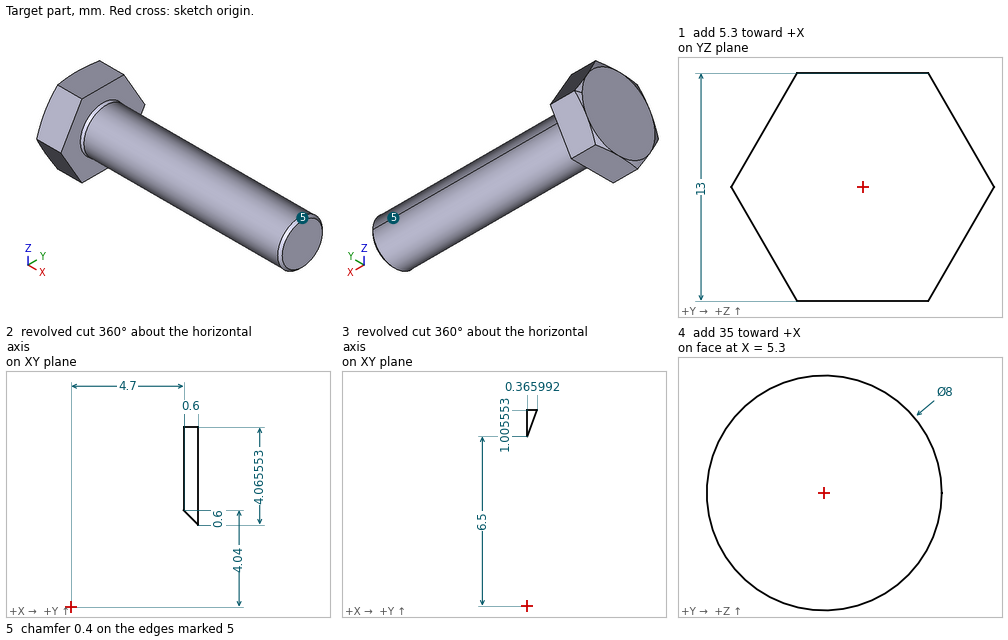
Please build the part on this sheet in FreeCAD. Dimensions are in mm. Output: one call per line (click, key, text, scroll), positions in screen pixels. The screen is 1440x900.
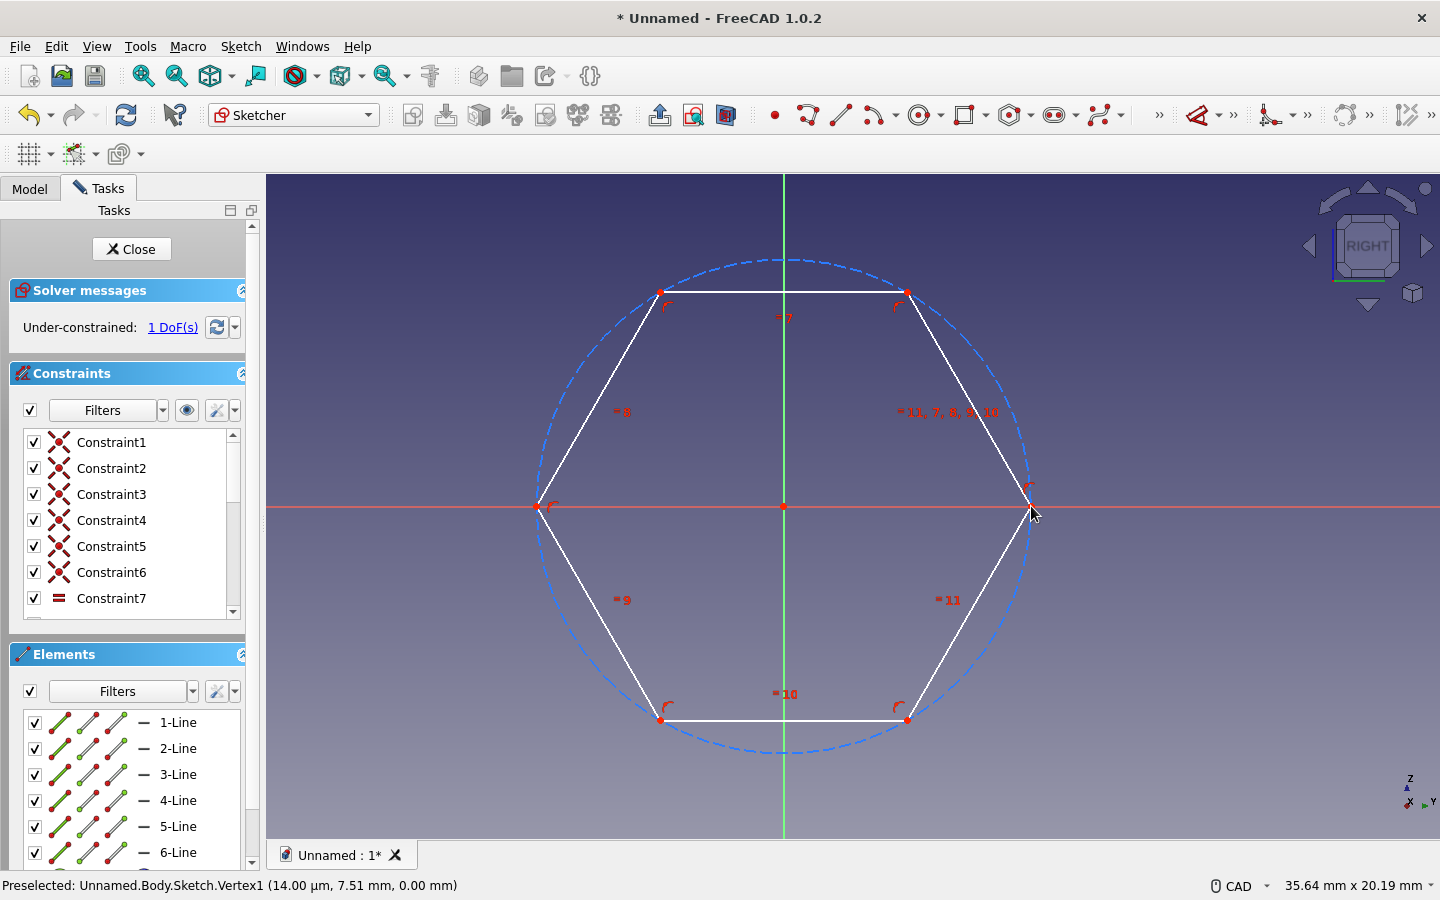
click(1196, 116)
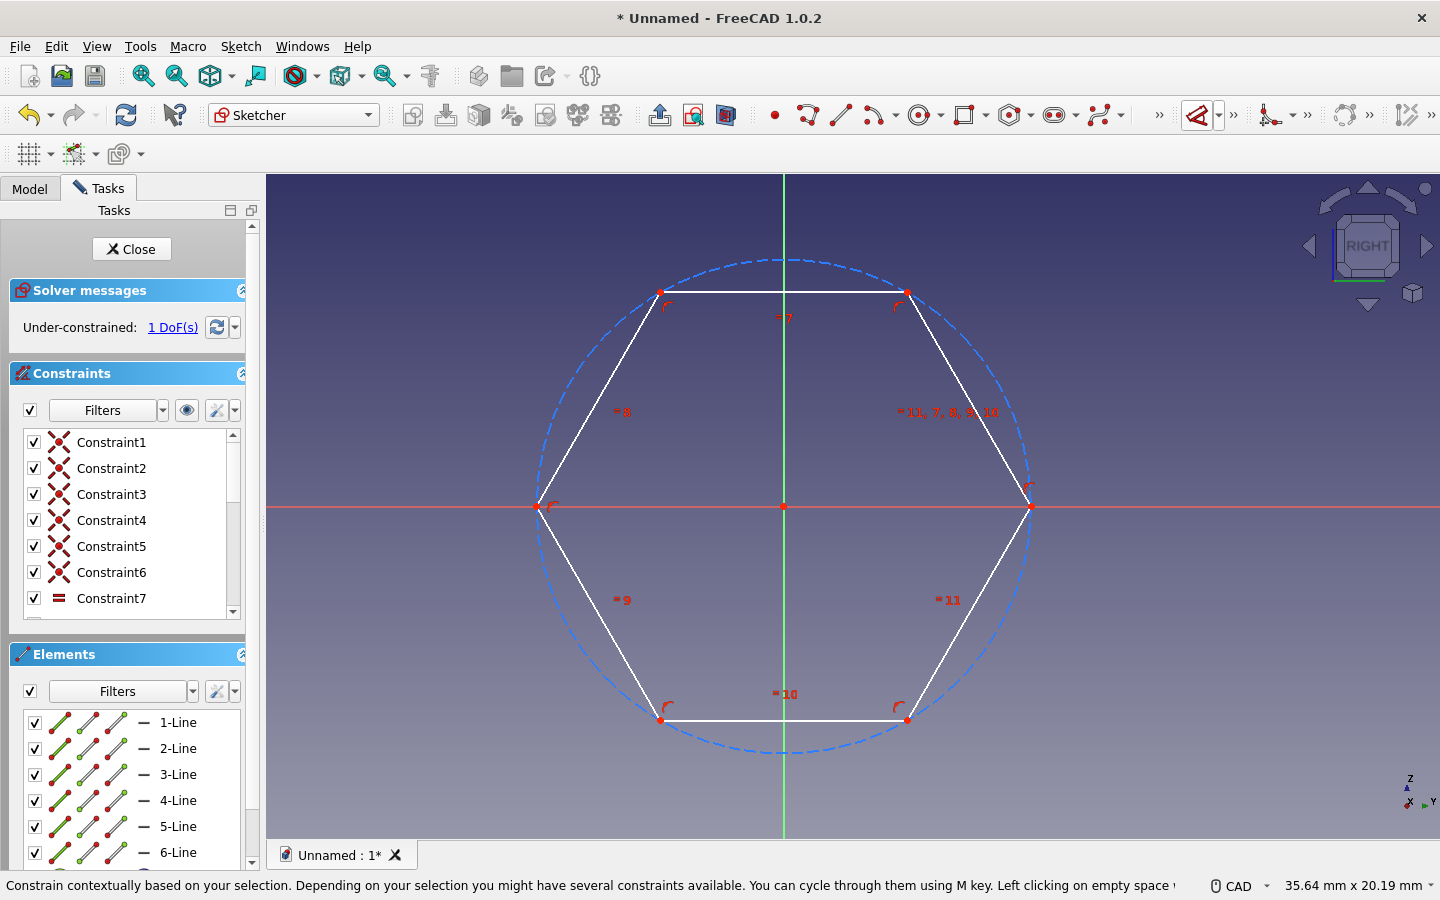
click(660, 721)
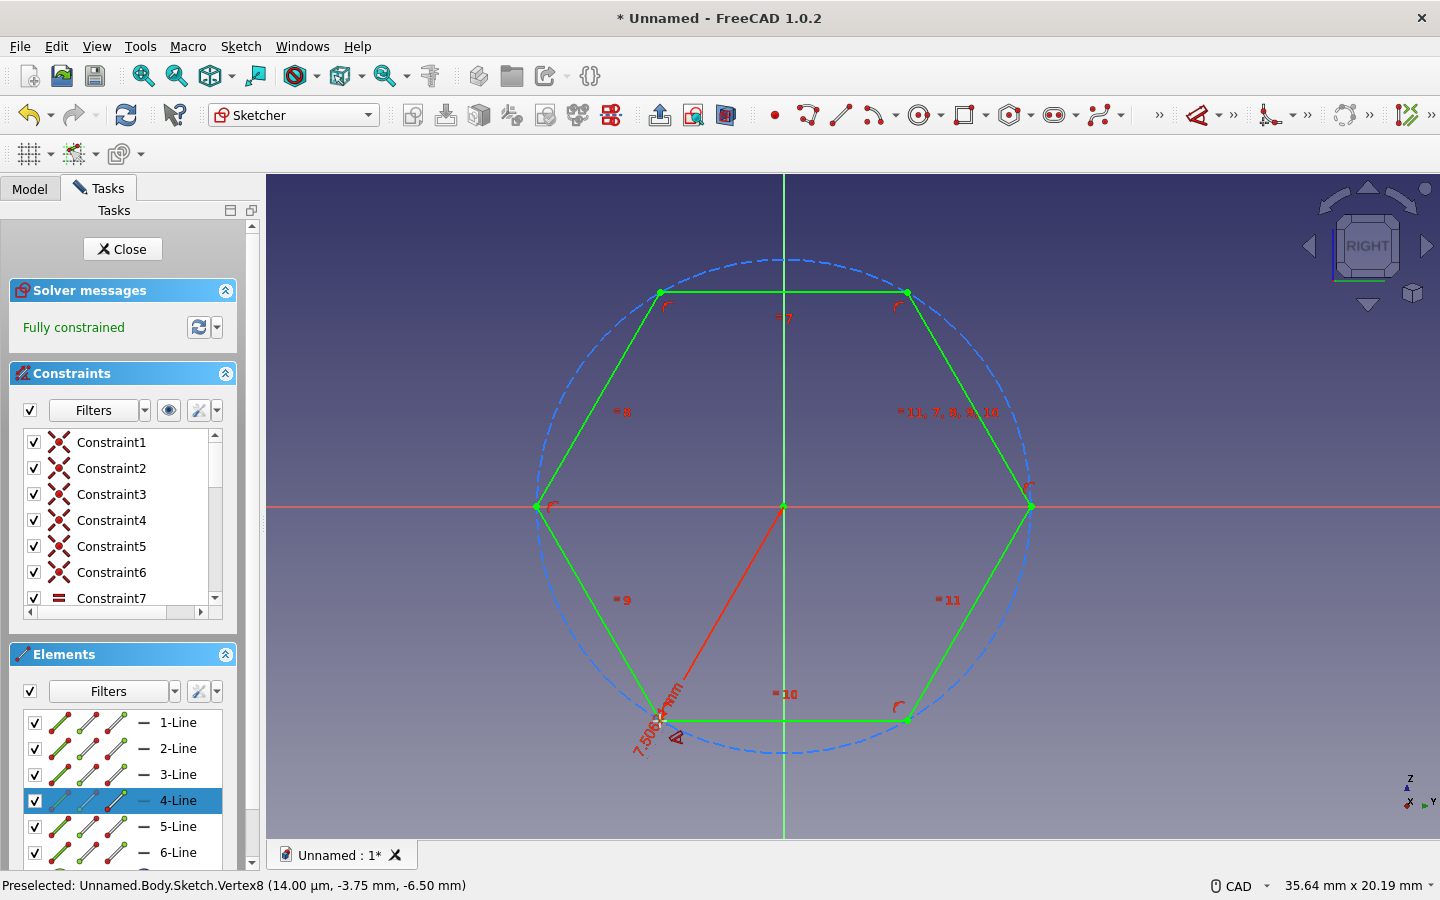
click(907, 292)
click(626, 408)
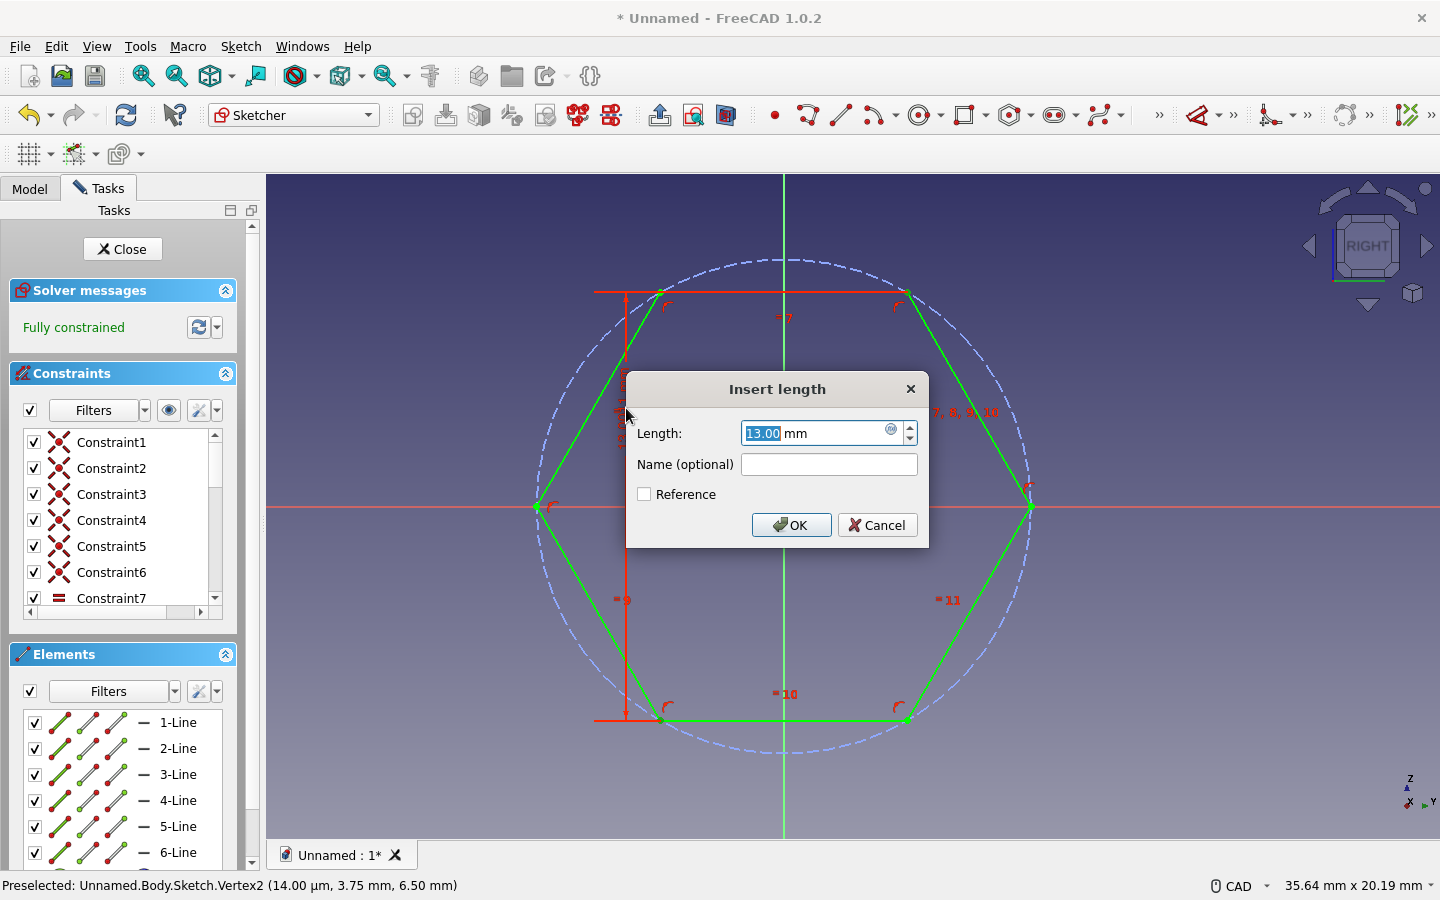
text(13)
key(Return)
key(Escape)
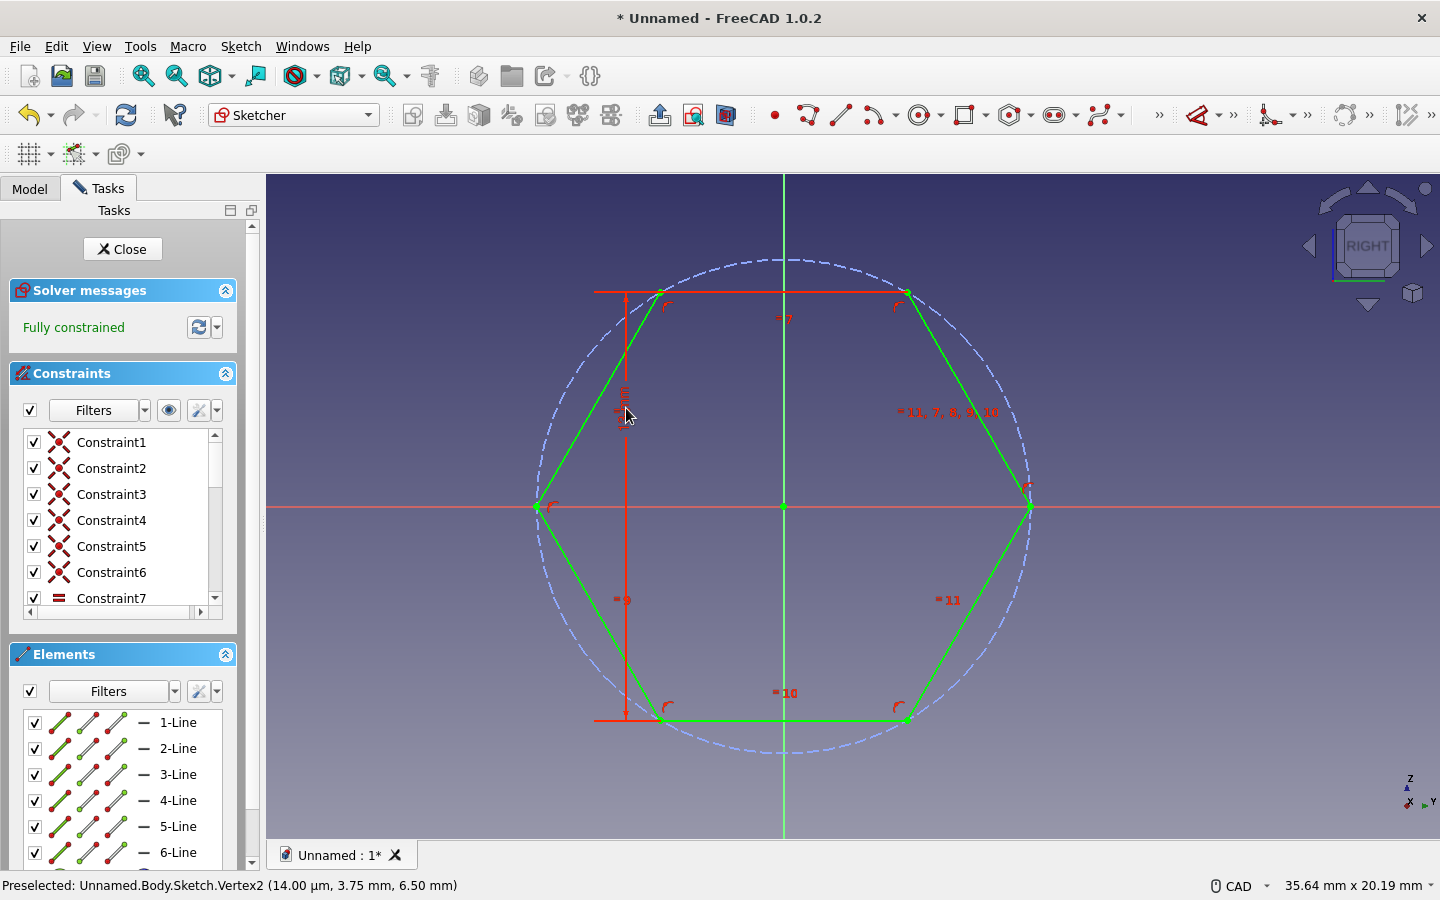
click(123, 249)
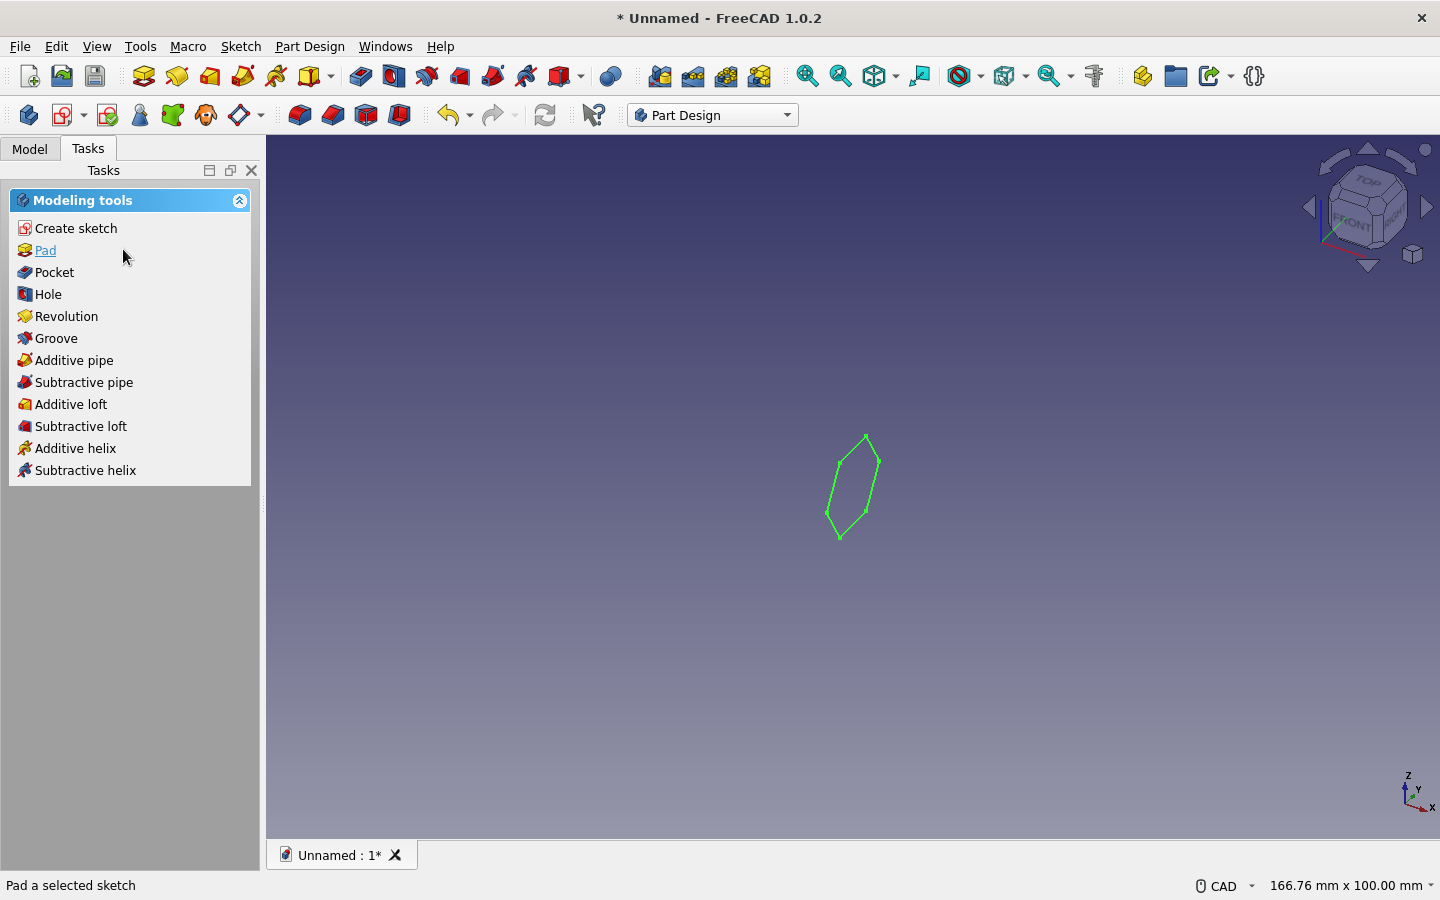
click(144, 76)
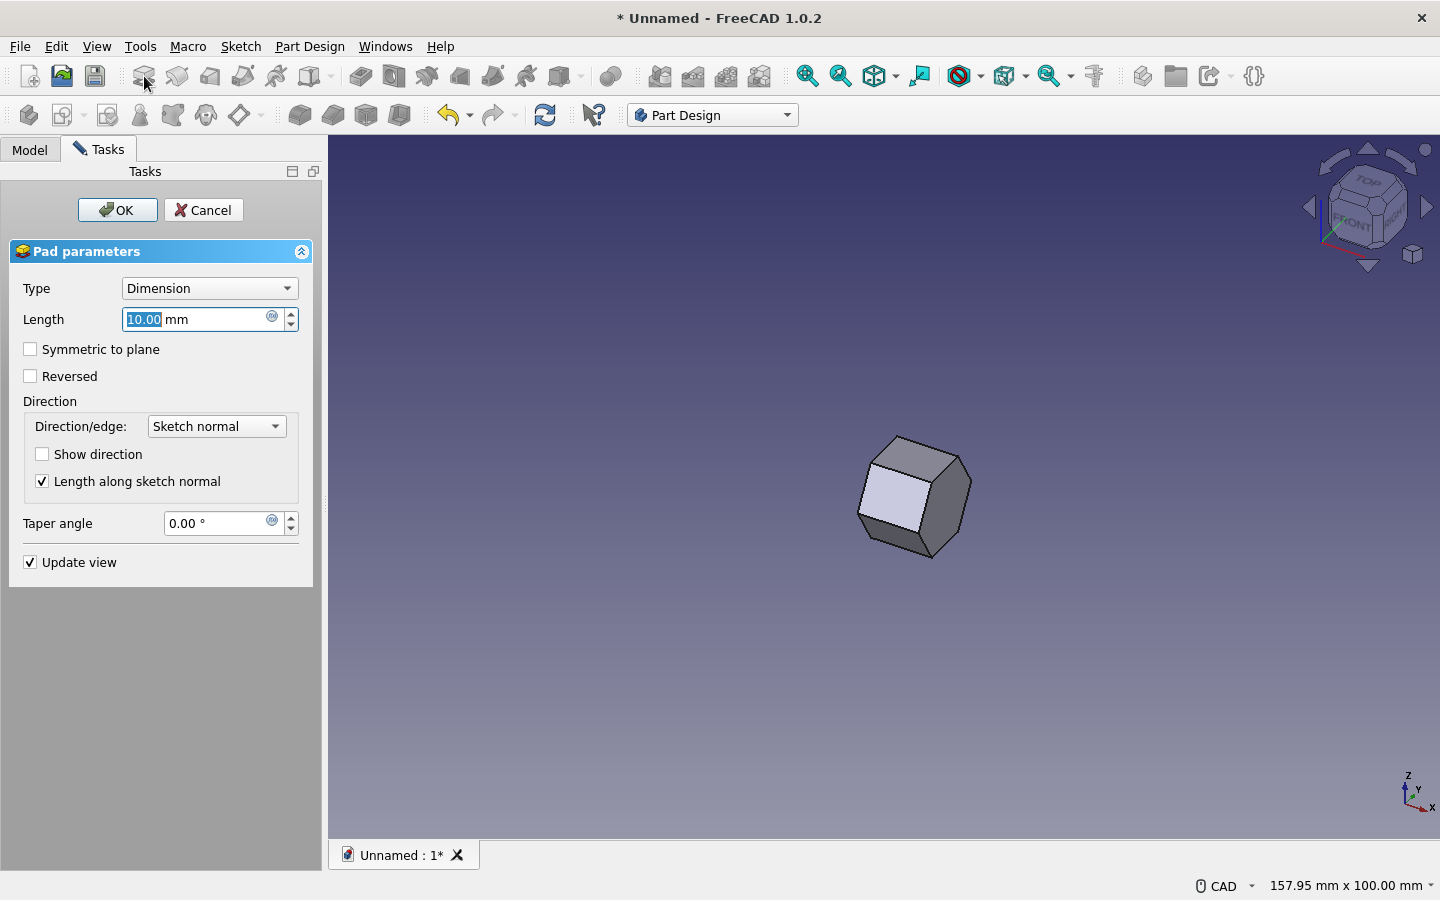
text(5.3)
key(Tab)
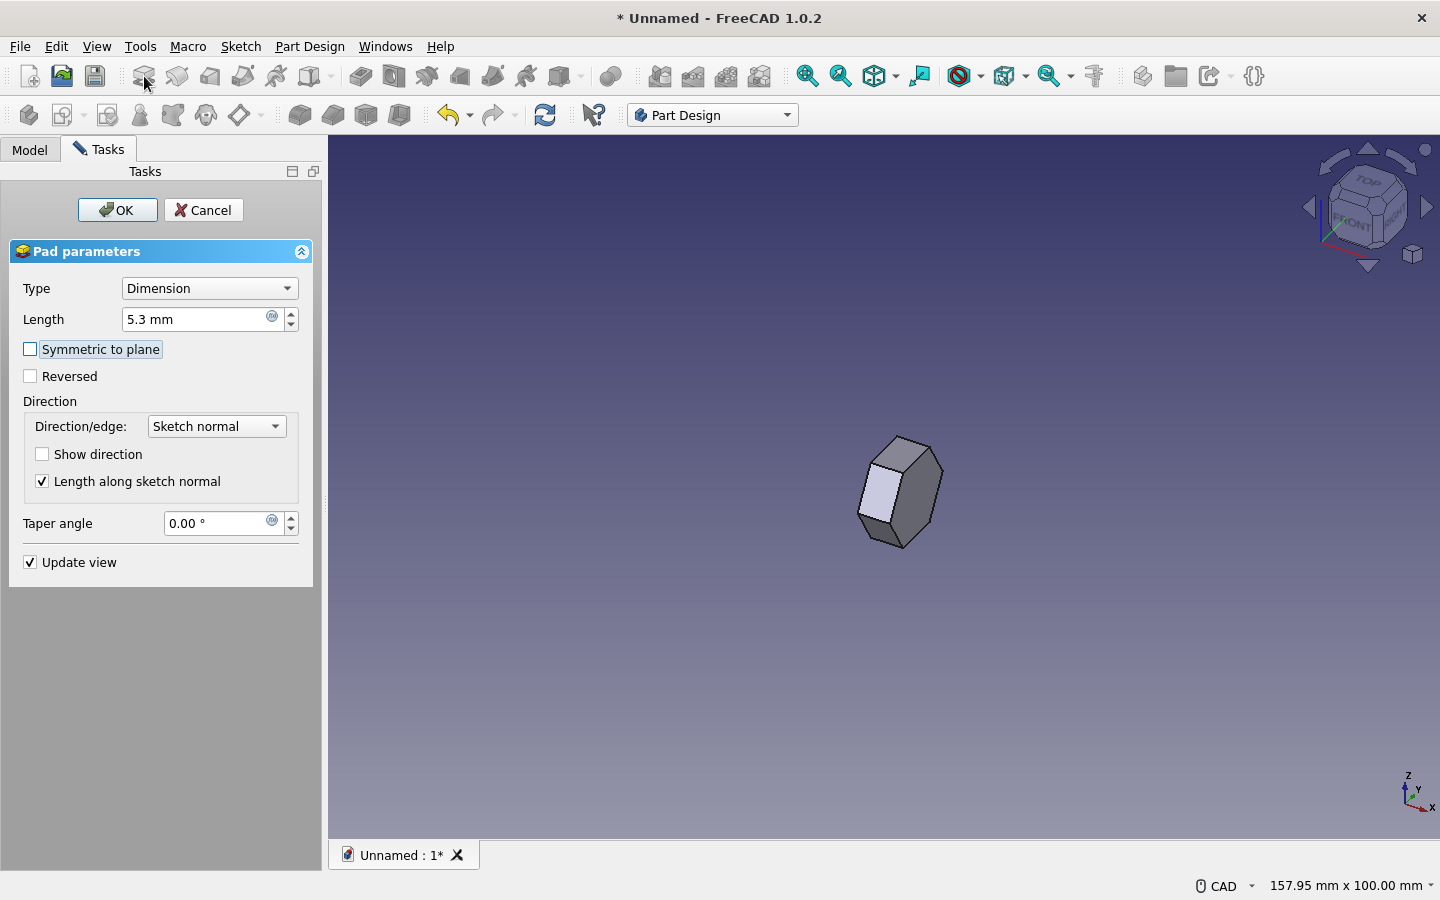
click(118, 210)